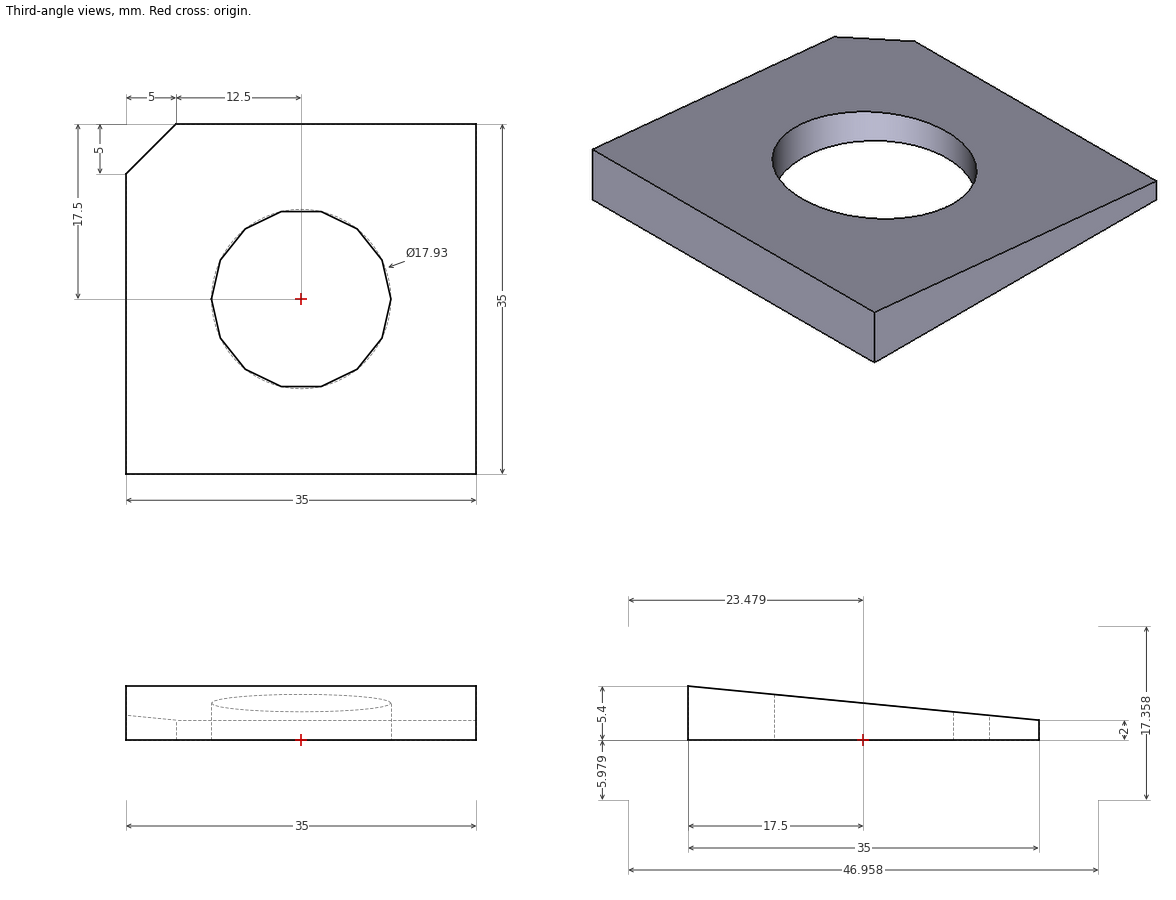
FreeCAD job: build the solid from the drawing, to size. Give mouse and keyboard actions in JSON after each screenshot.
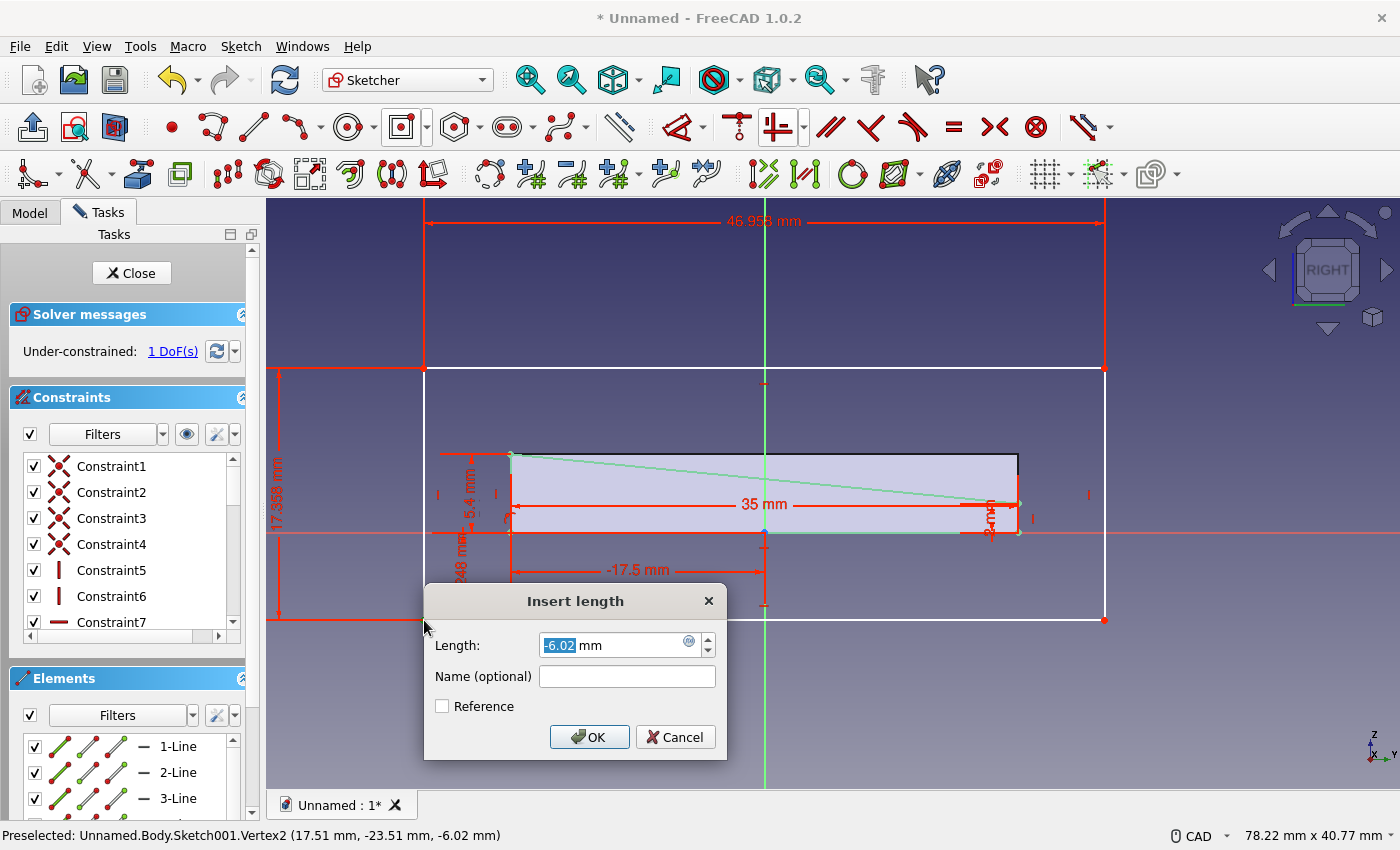
{"action": "type", "text": "-5.979"}
{"action": "key", "text": "Return"}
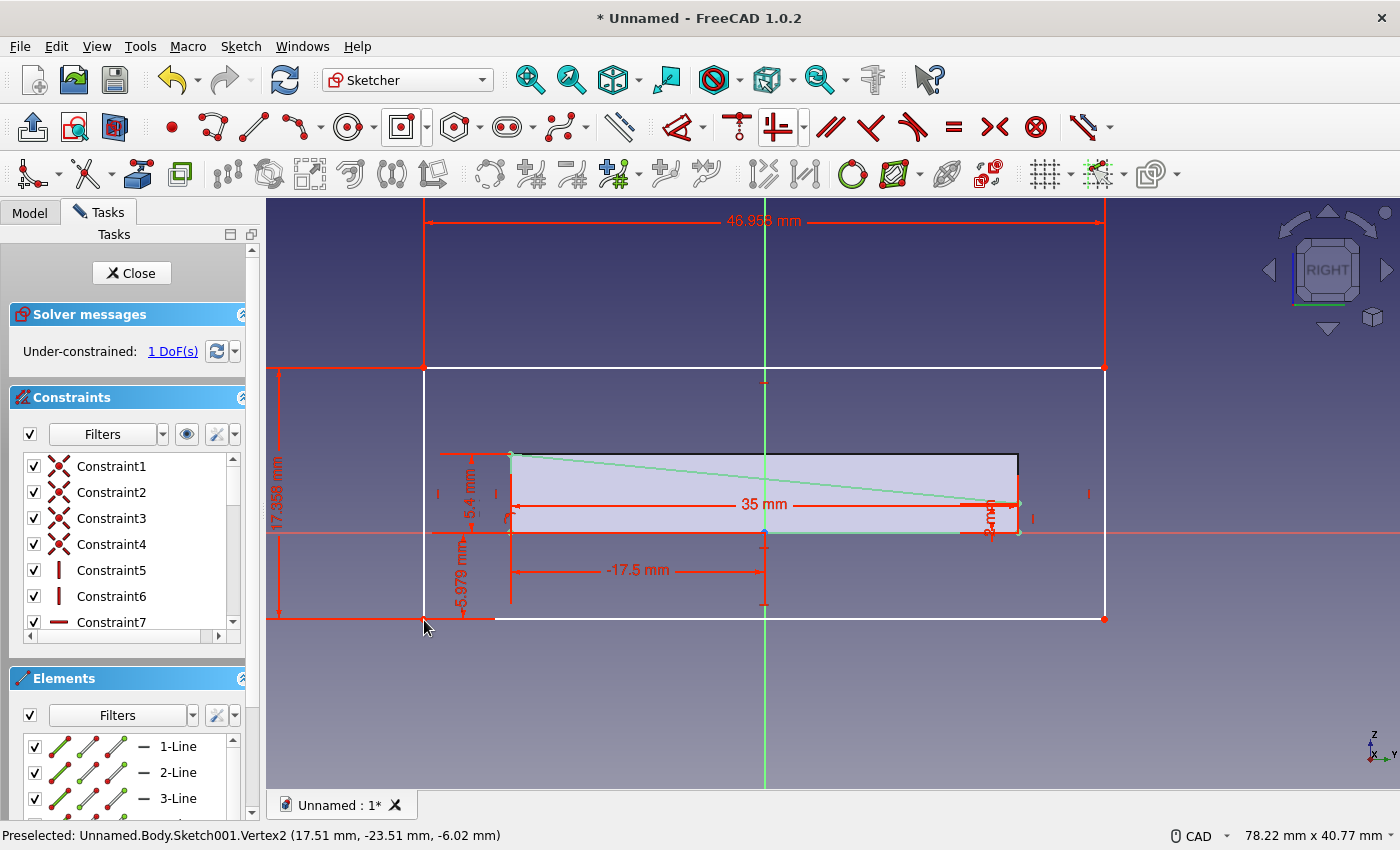
{"action": "left_click", "coordinate": [424, 368]}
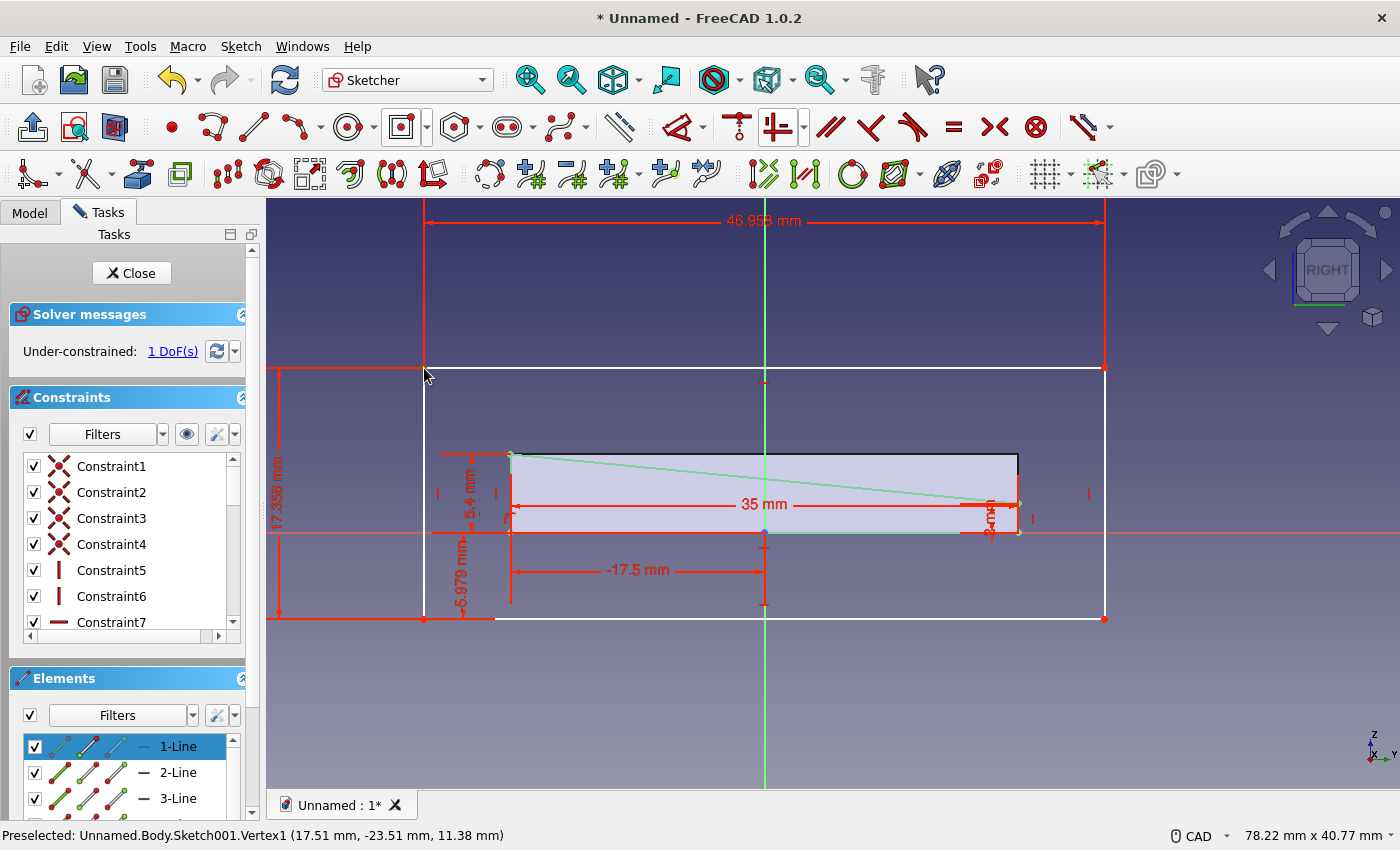
{"action": "key", "text": "l"}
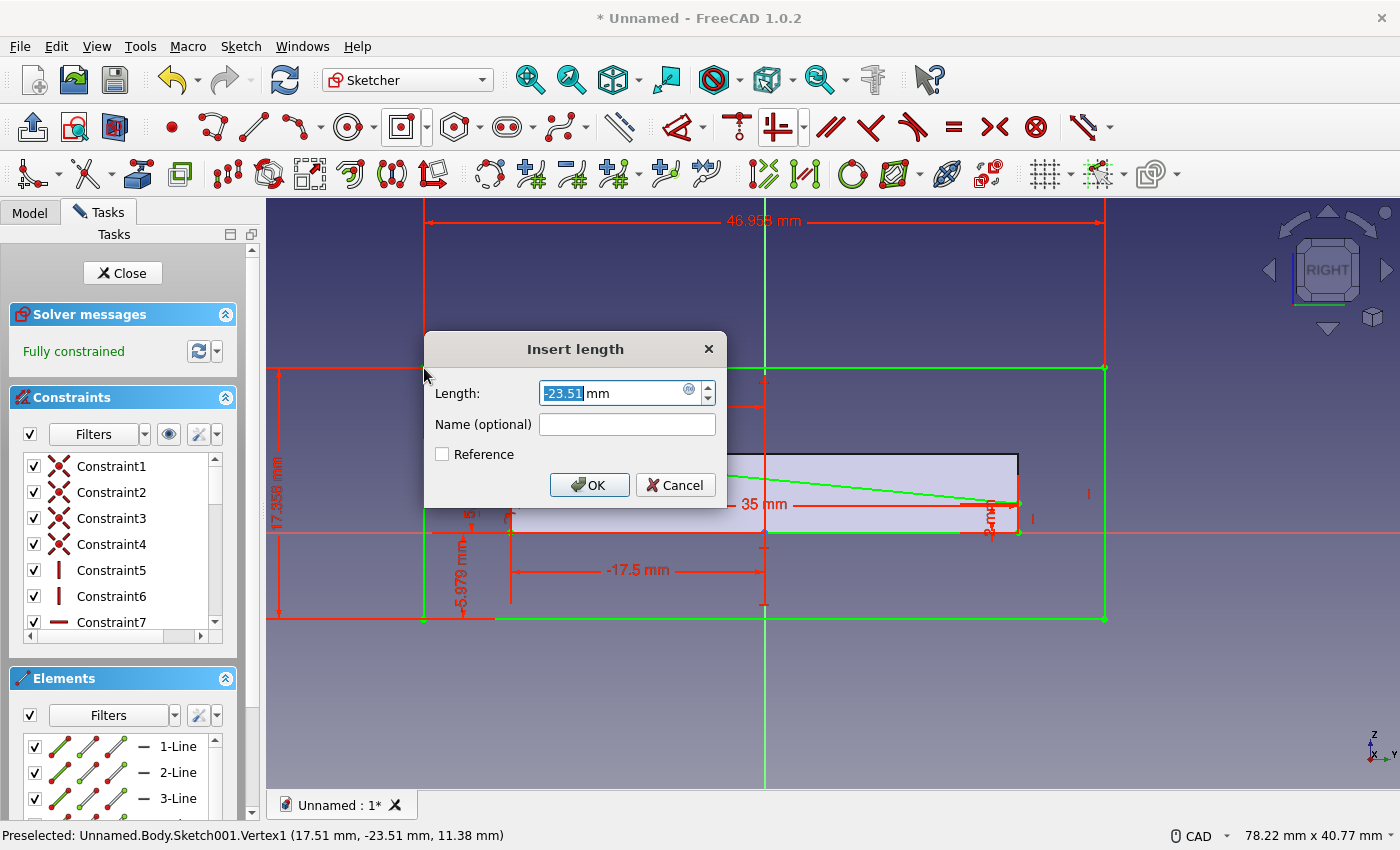
{"action": "type", "text": "-23.479"}
{"action": "key", "text": "Return"}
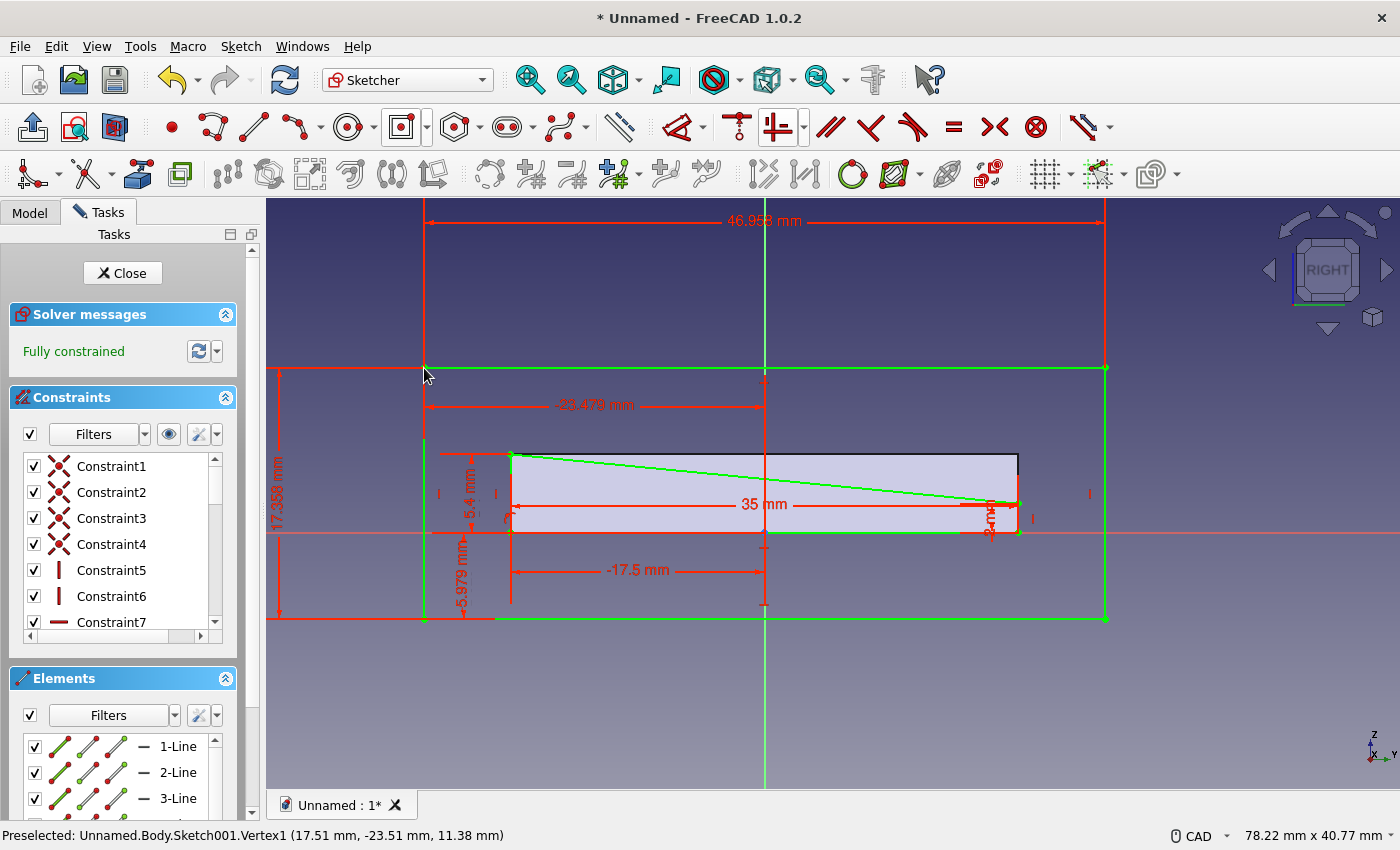
{"action": "left_click", "coordinate": [123, 273]}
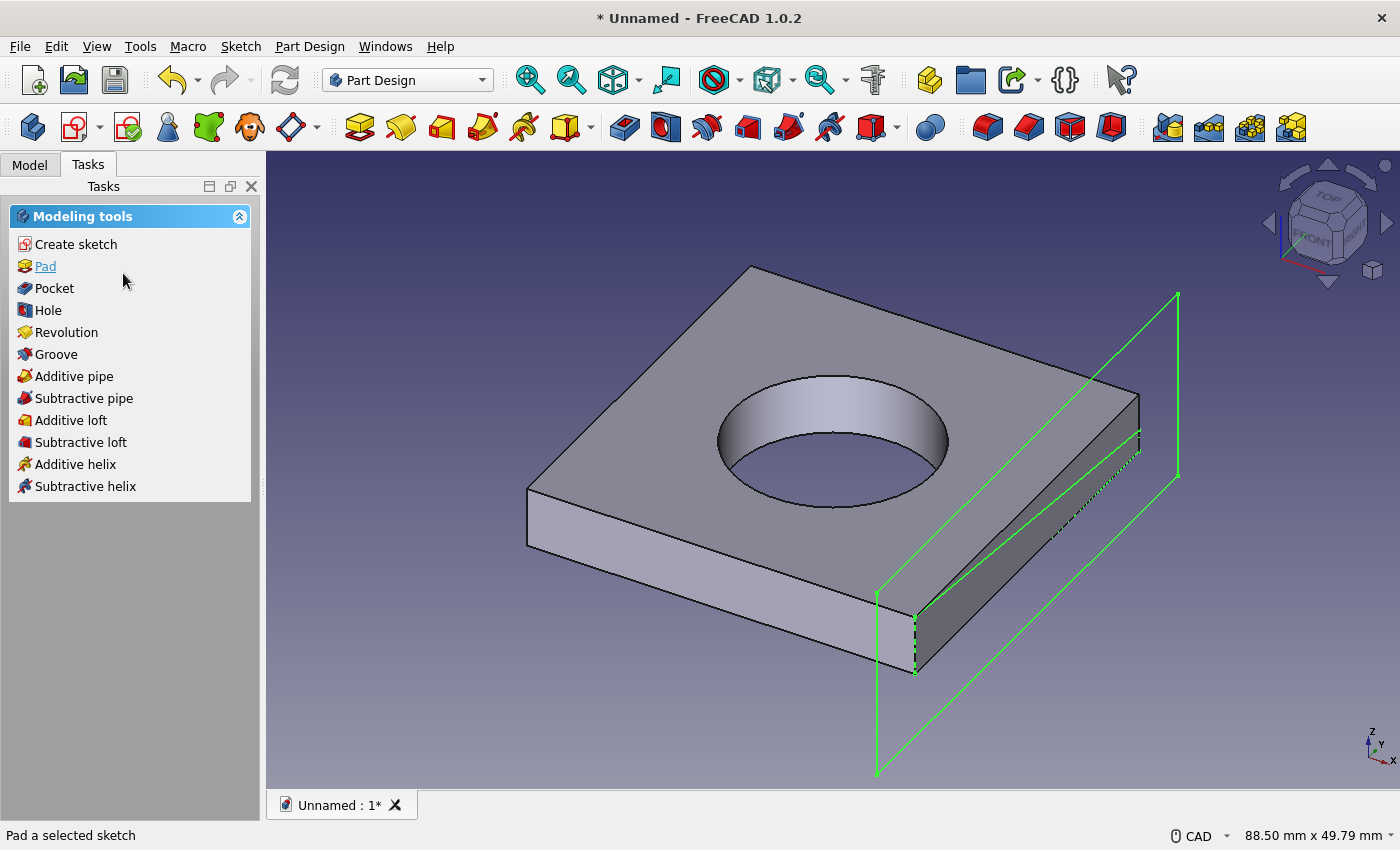
{"action": "left_click", "coordinate": [625, 128]}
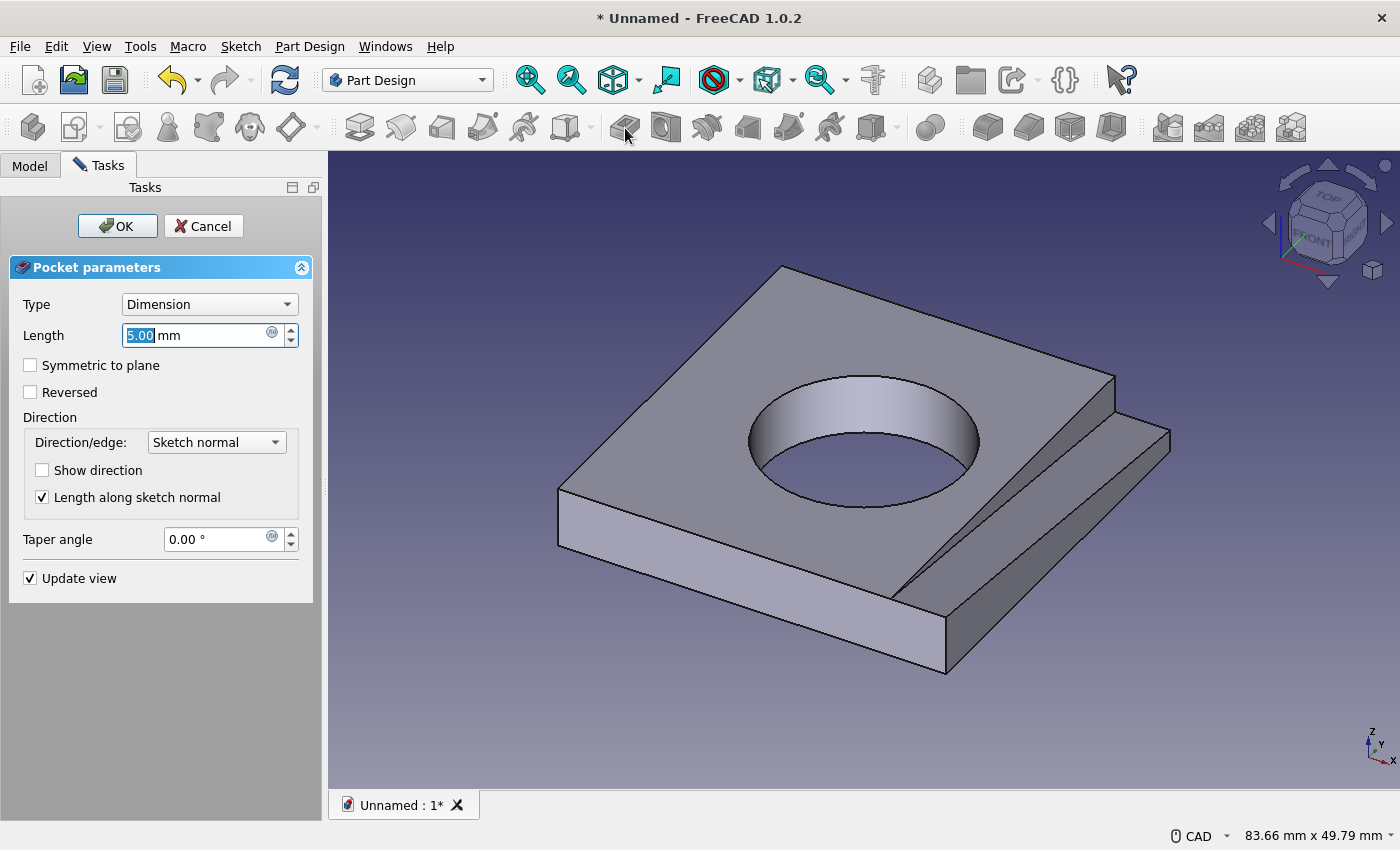
{"action": "type", "text": "35"}
{"action": "key", "text": "Tab"}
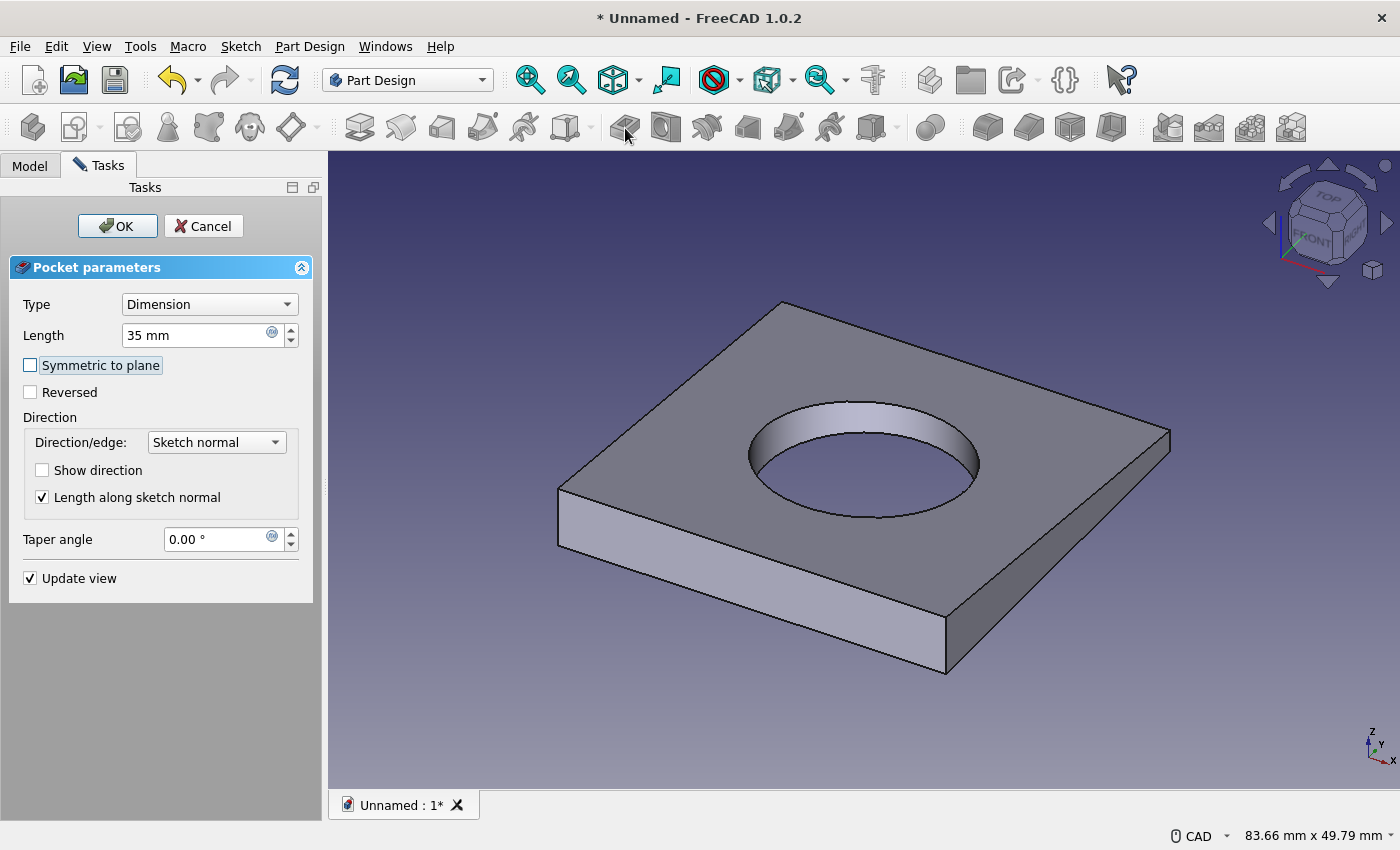
{"action": "left_click", "coordinate": [118, 226]}